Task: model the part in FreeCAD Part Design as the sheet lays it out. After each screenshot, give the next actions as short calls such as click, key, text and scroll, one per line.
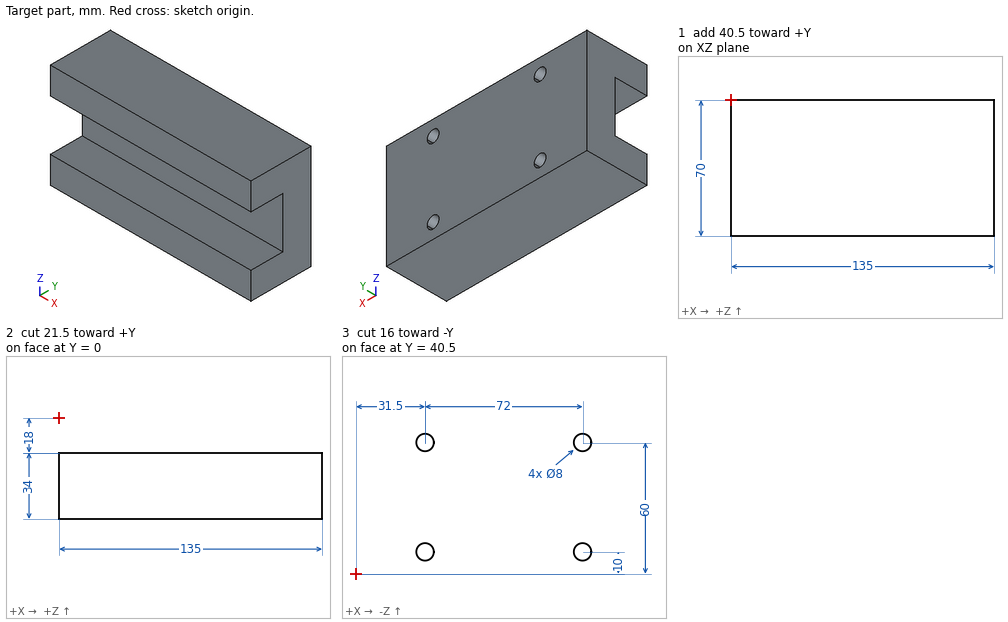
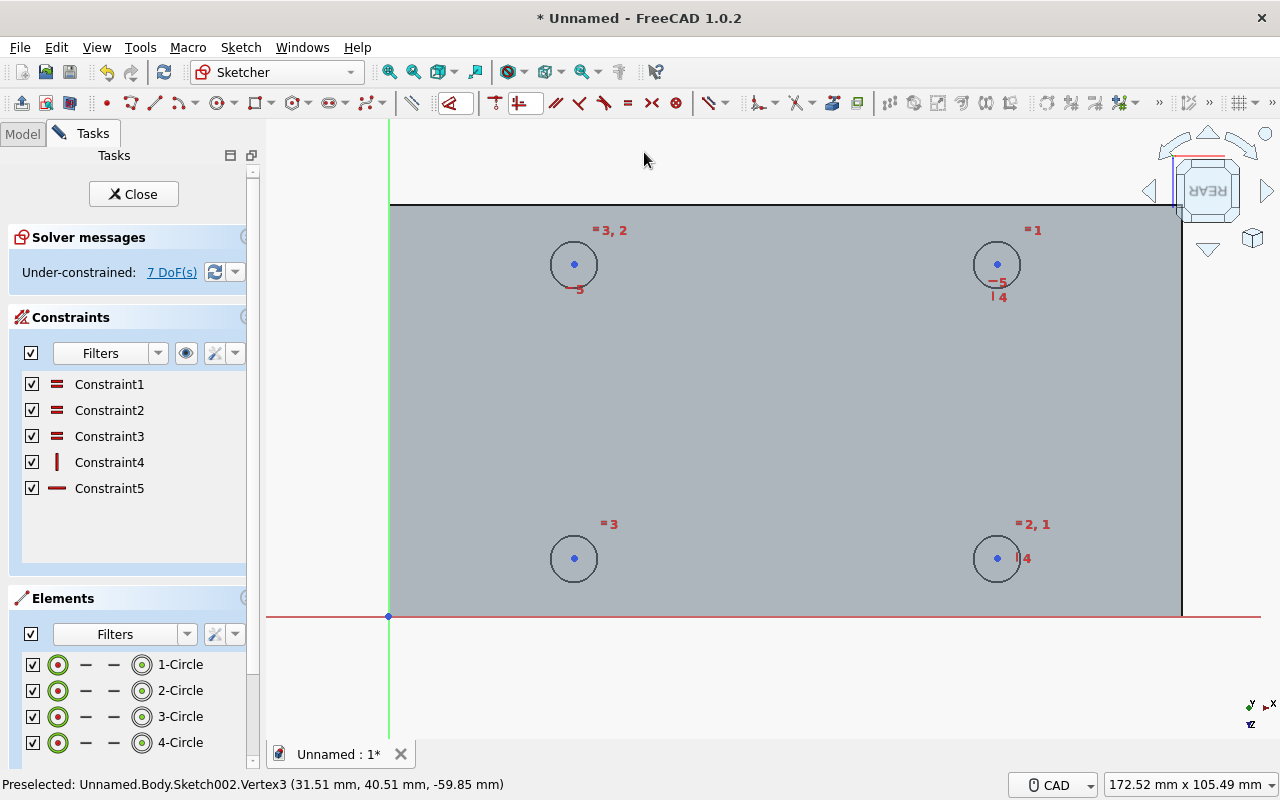
click(574, 265)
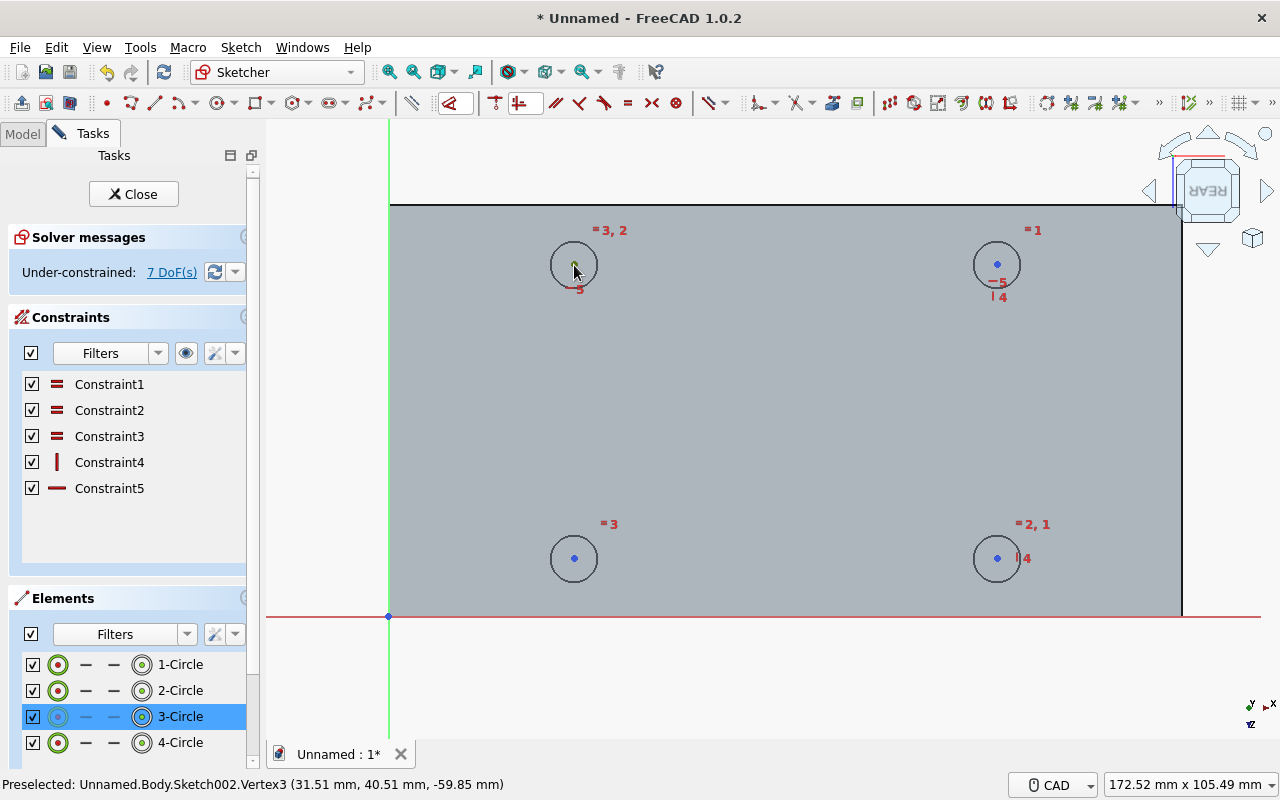
click(574, 559)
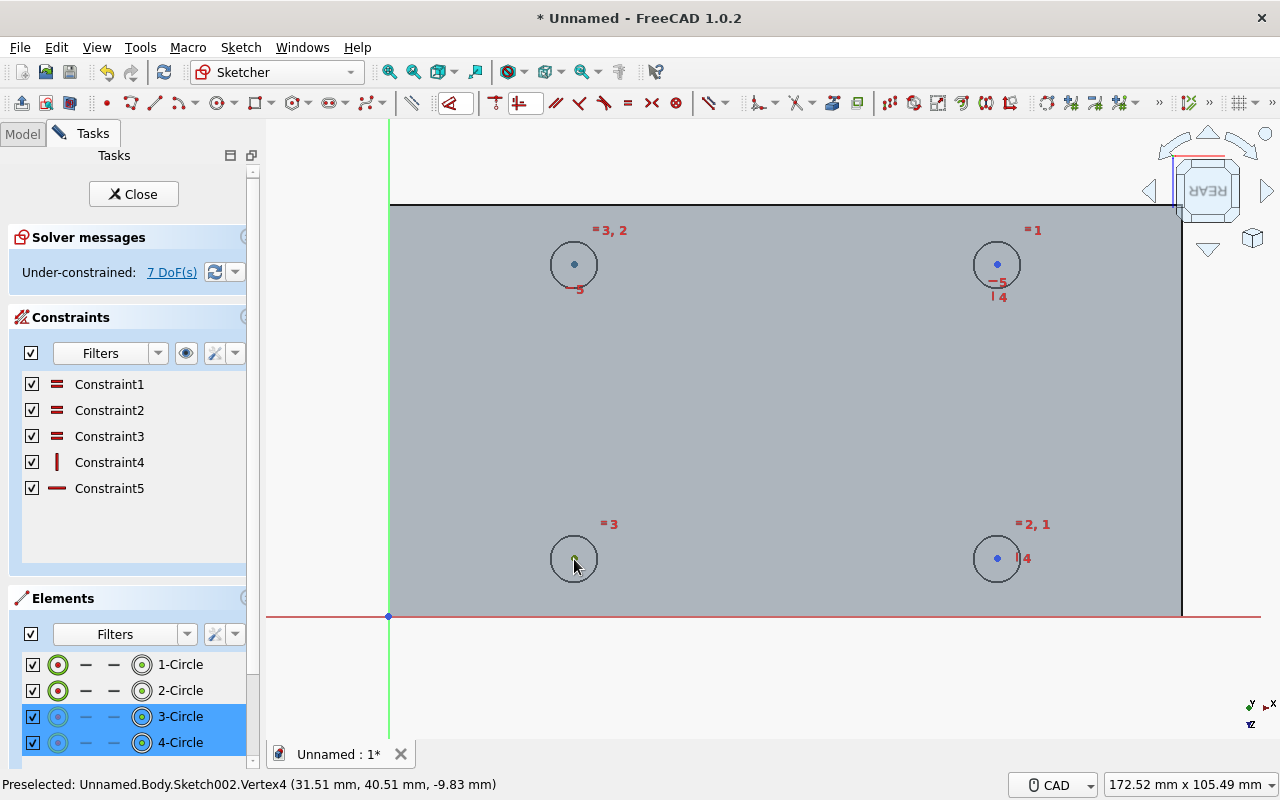
key(v)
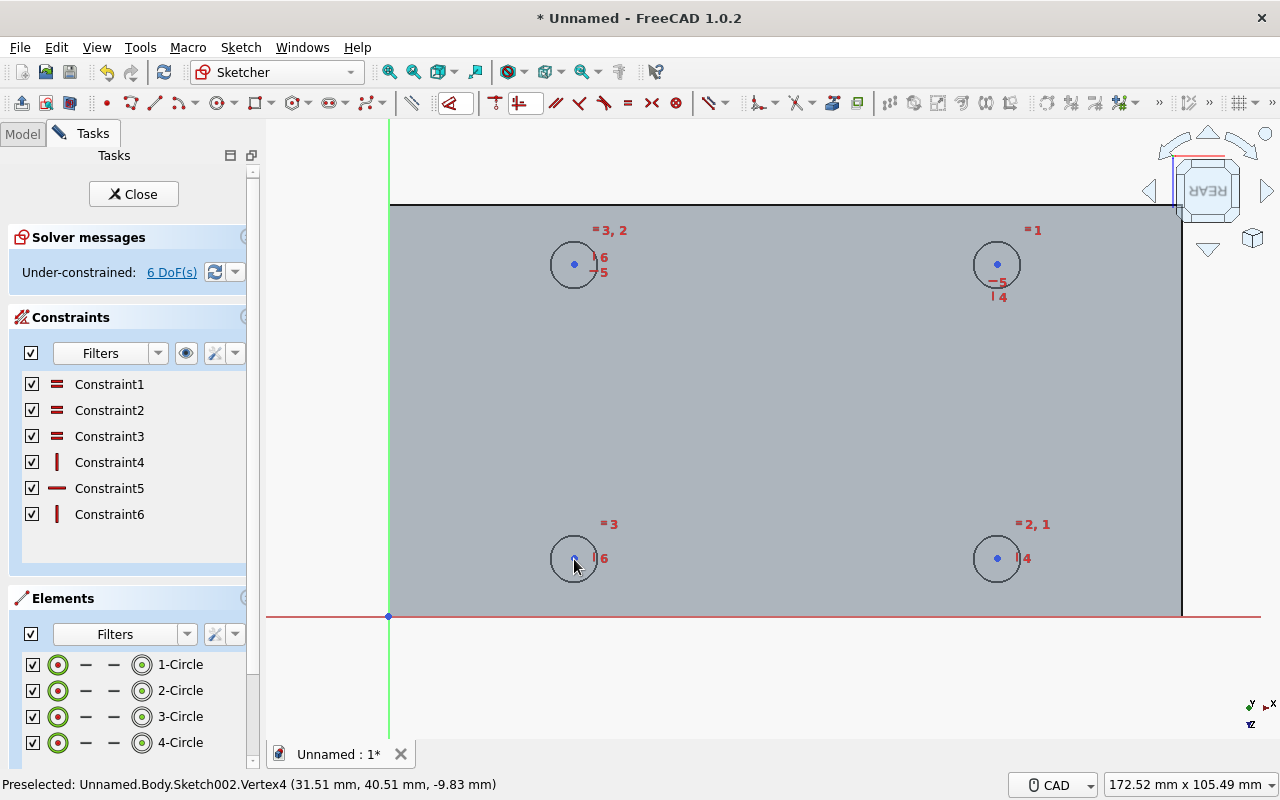
click(997, 559)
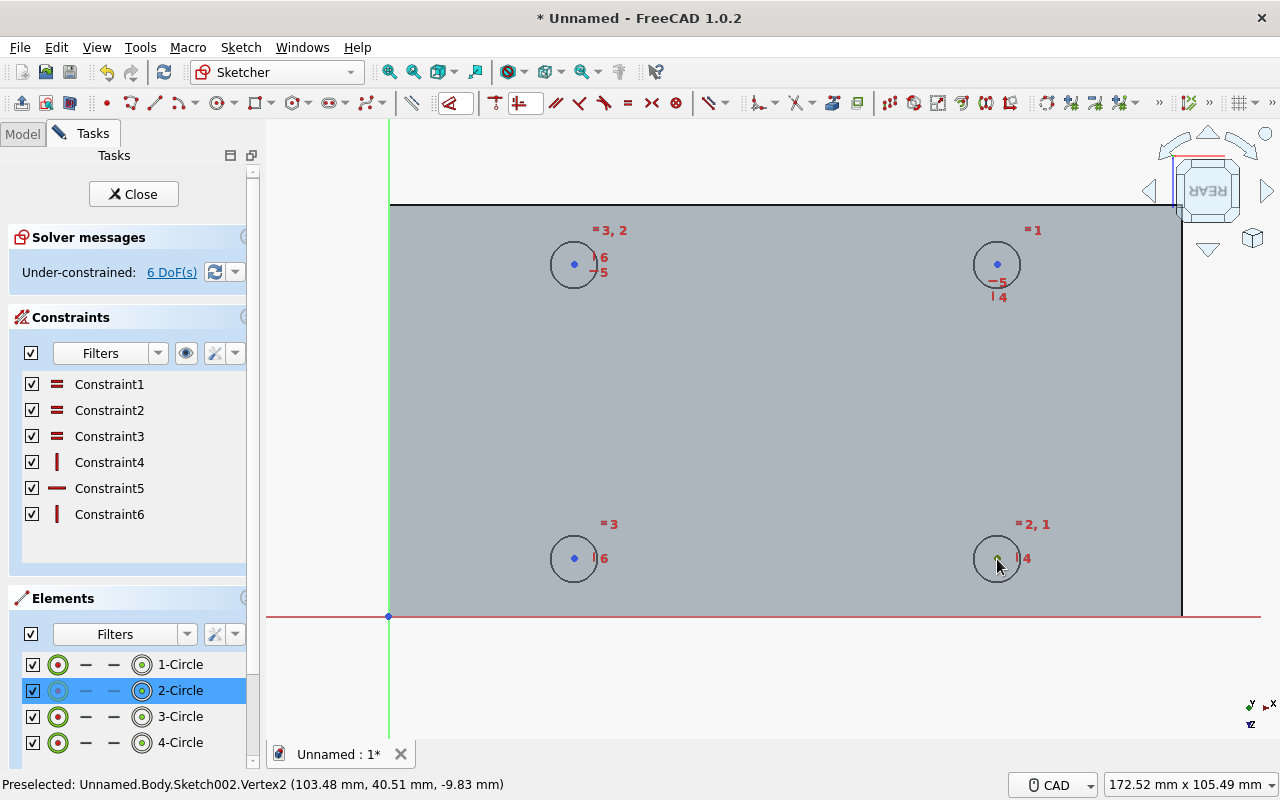
click(574, 559)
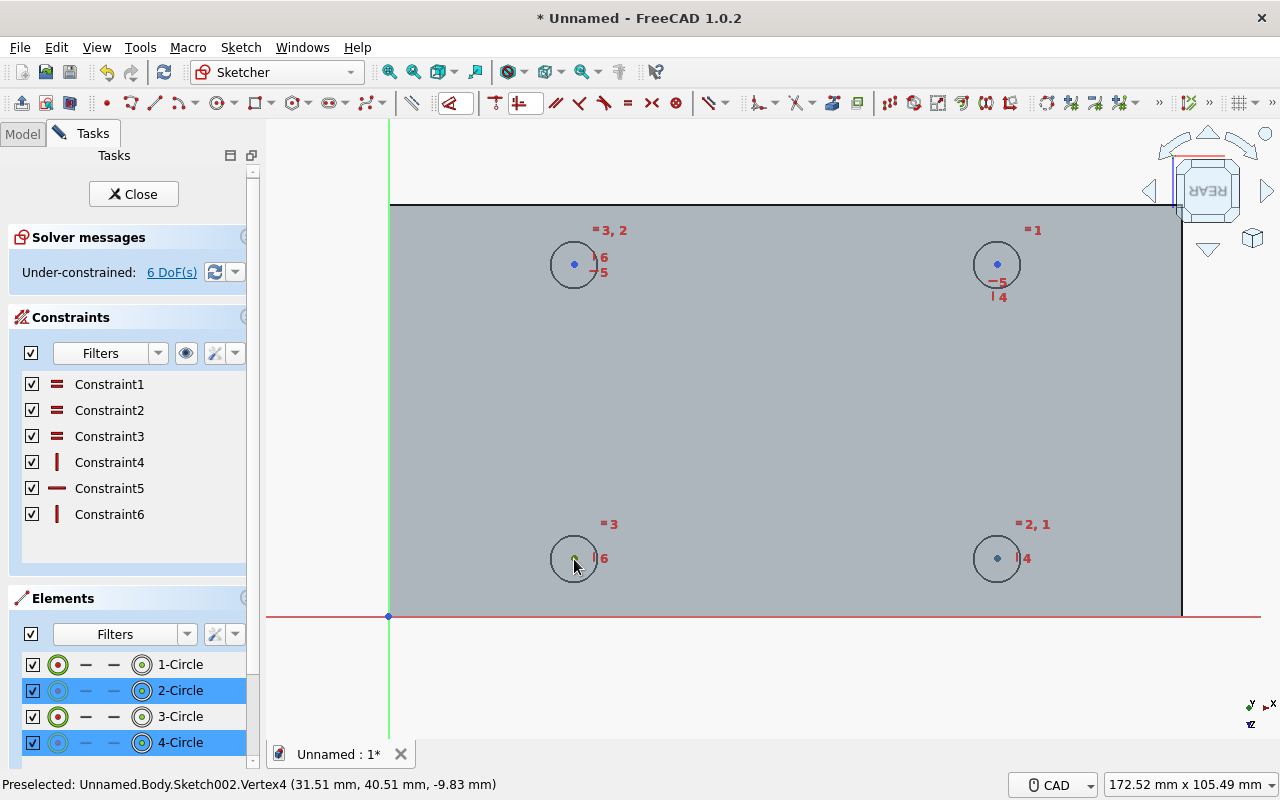
key(h)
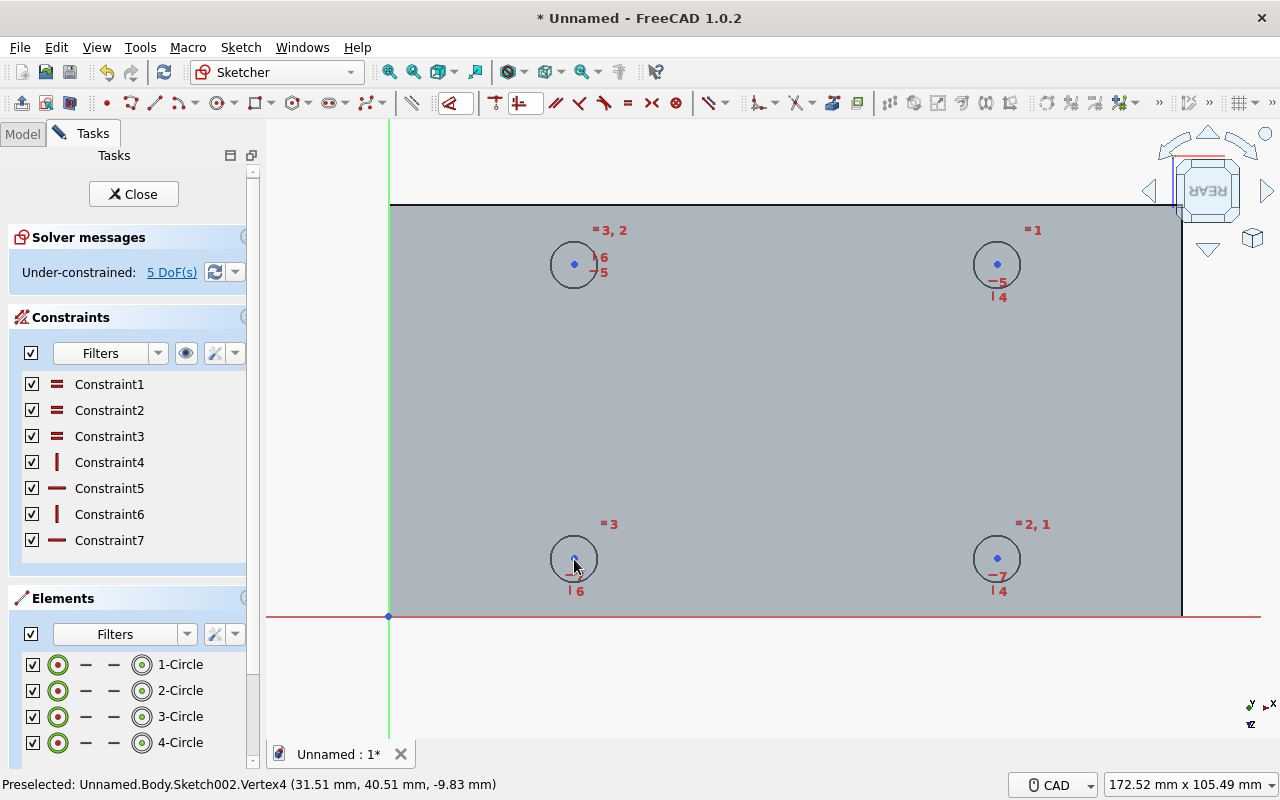
click(1013, 248)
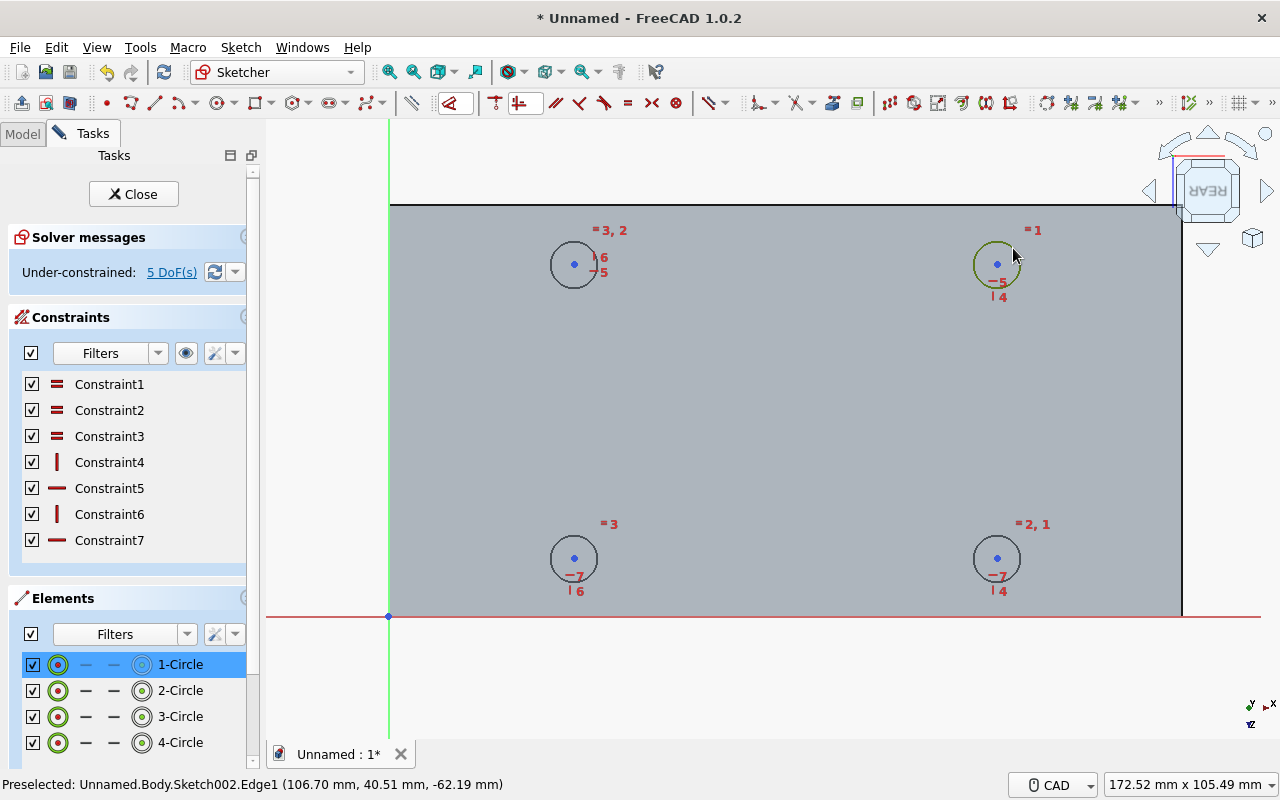
key(k)
key(o)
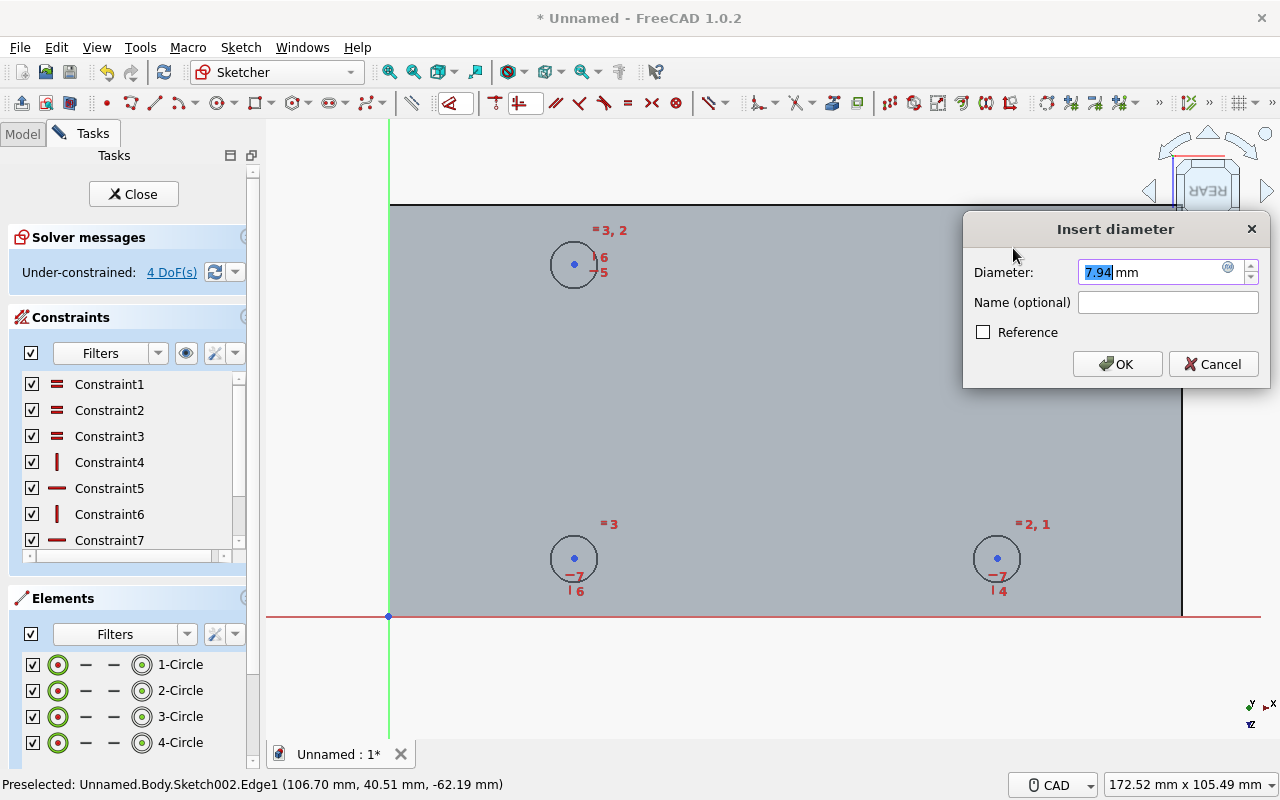
text(8)
key(Return)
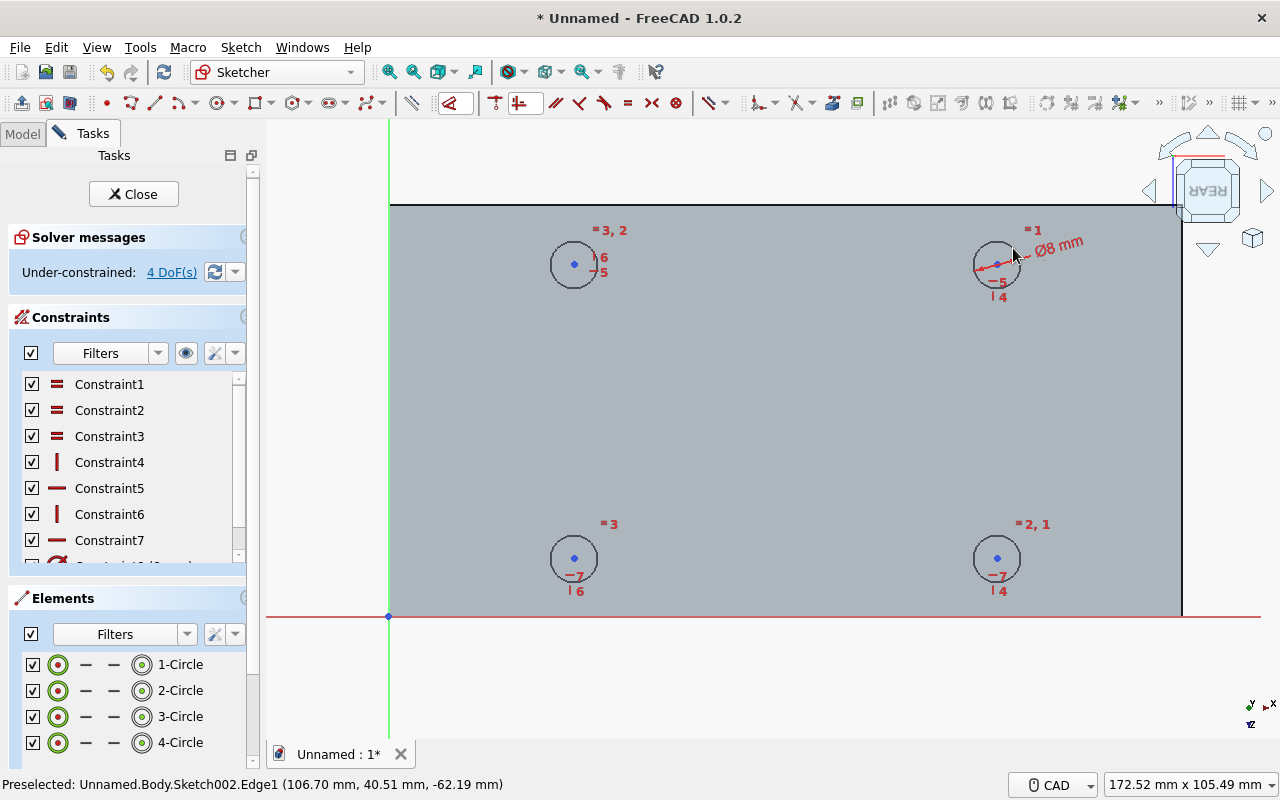
click(997, 265)